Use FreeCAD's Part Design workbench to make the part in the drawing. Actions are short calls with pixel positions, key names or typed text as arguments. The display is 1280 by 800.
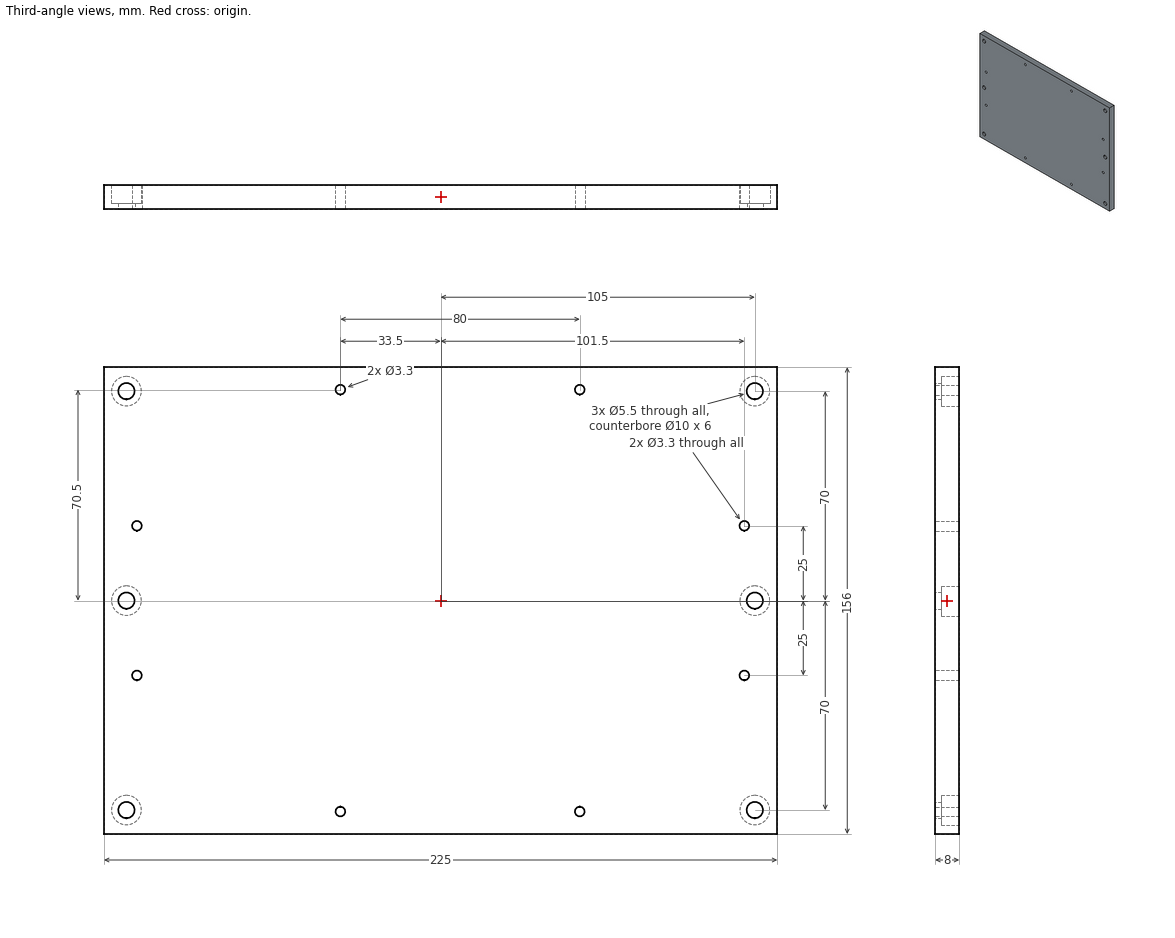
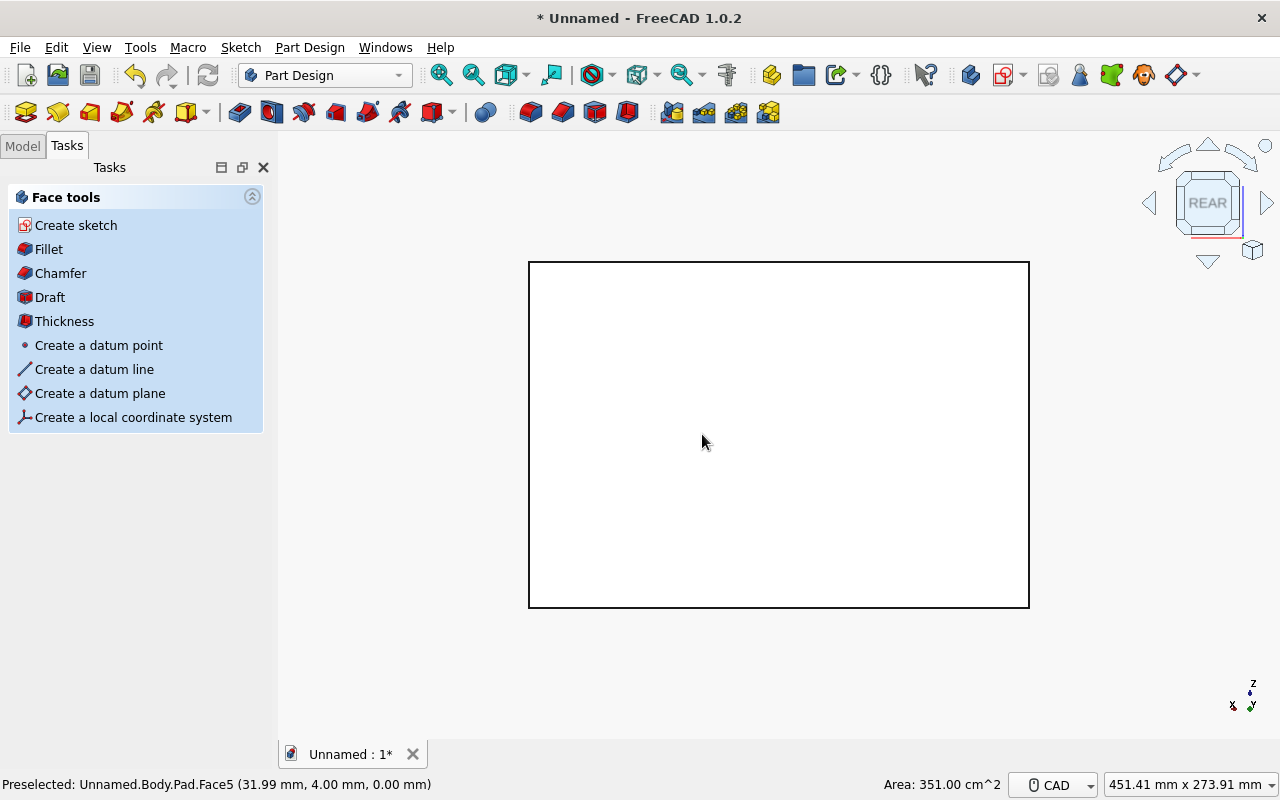
click(1004, 76)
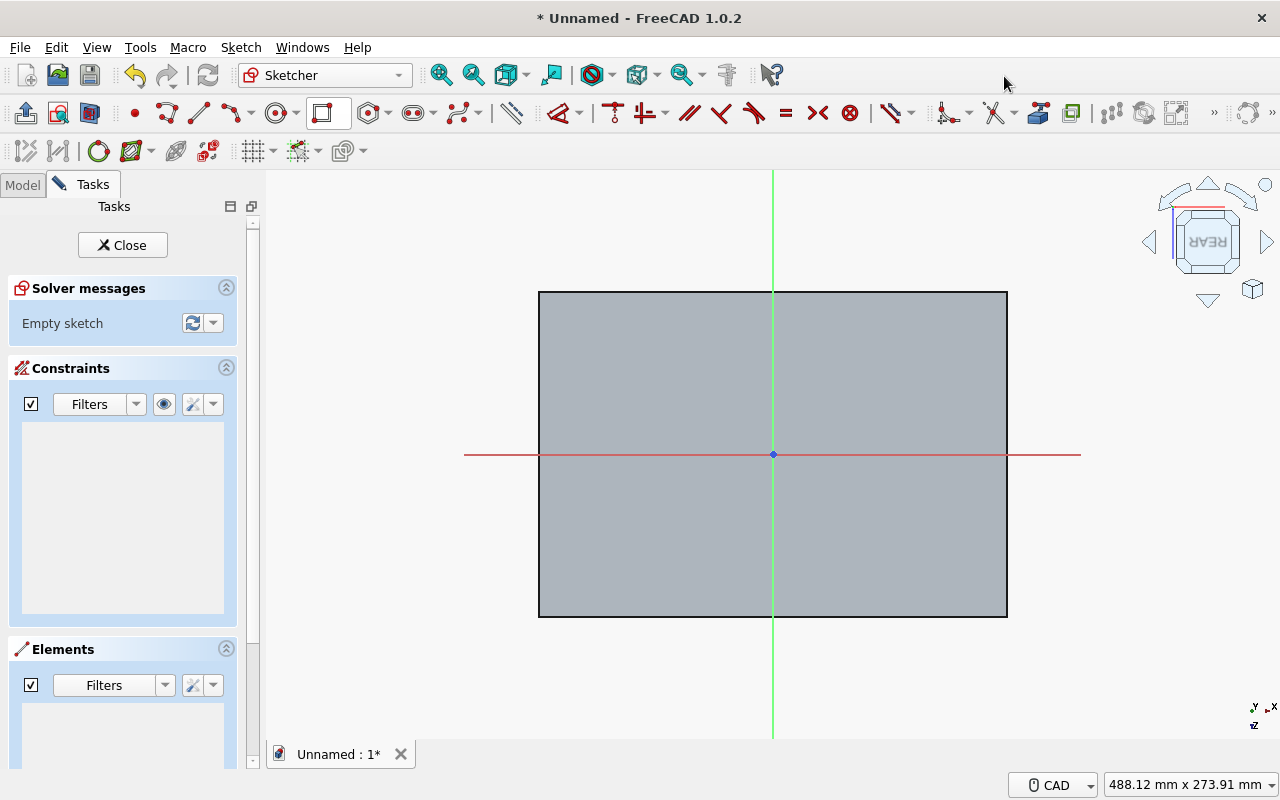
key(g)
key(c)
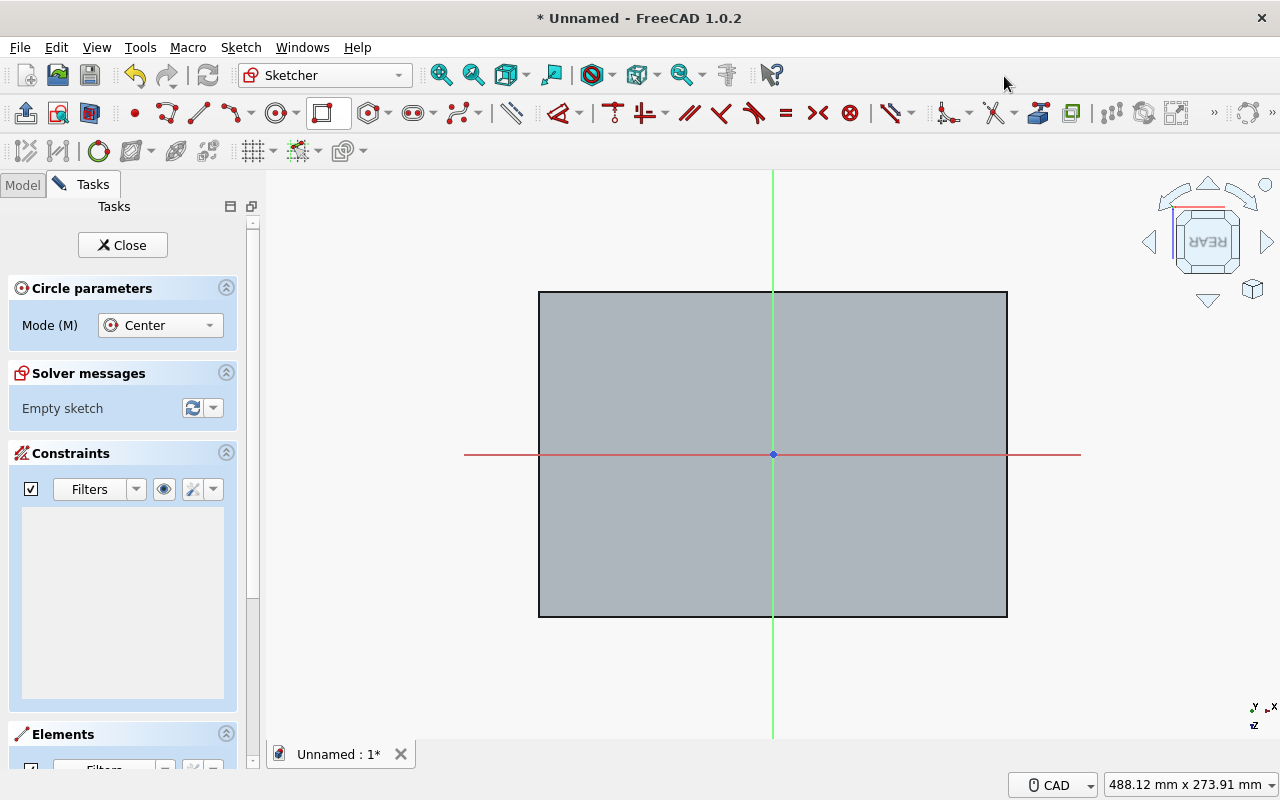
scroll(991, 600, up, 7)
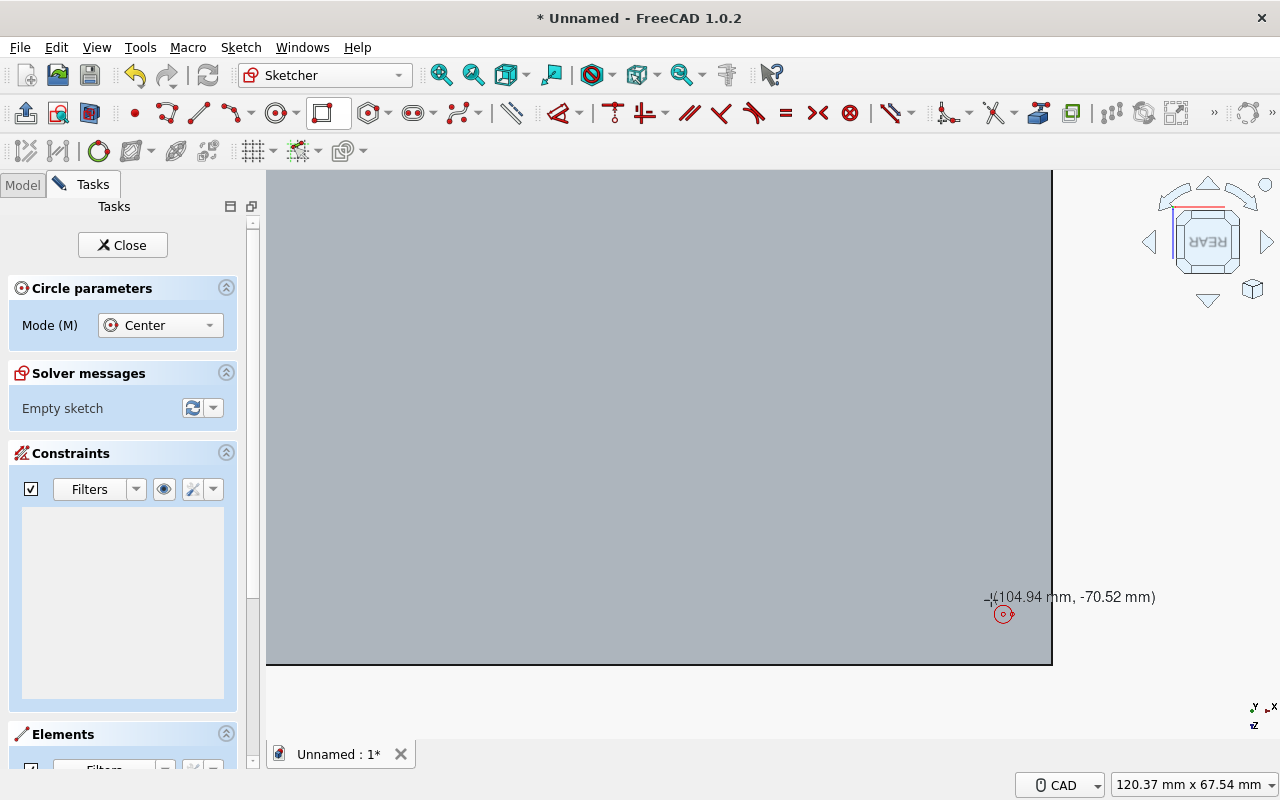
scroll(767, 647, down, 6)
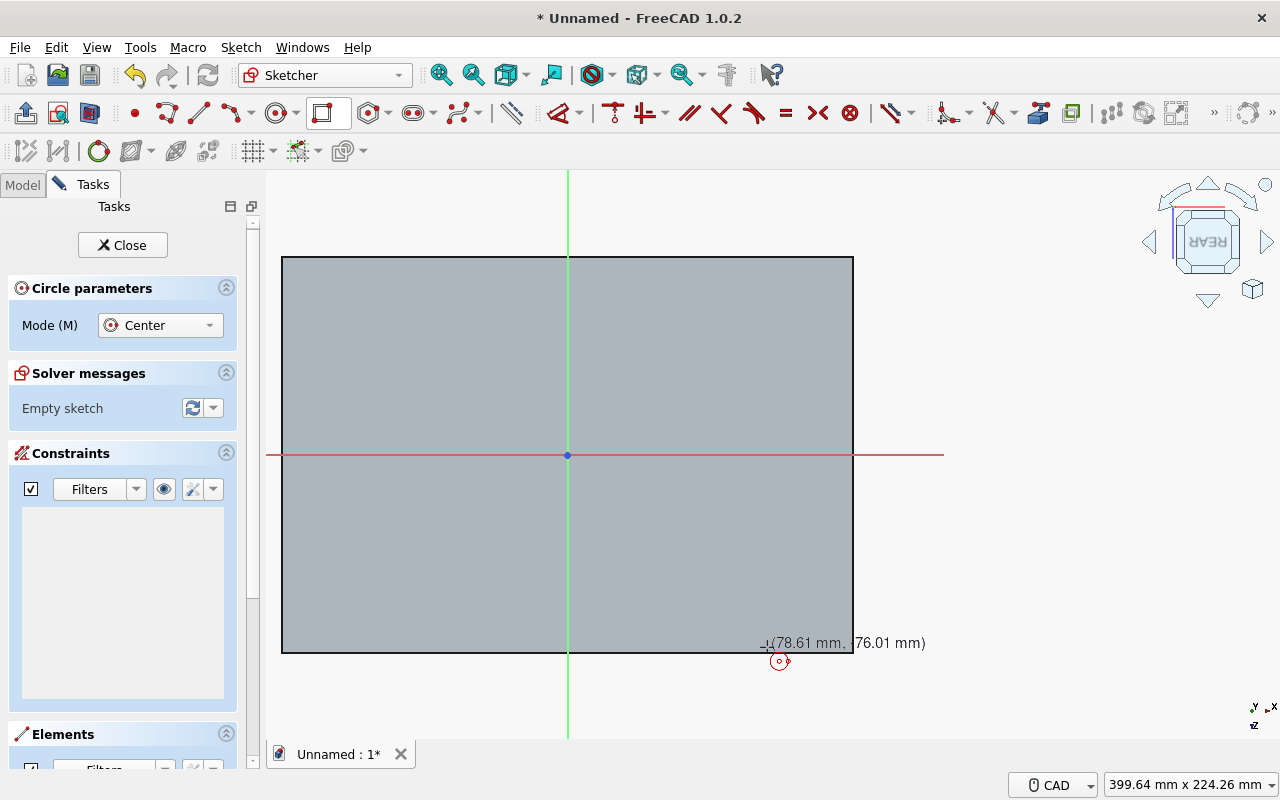
click(834, 633)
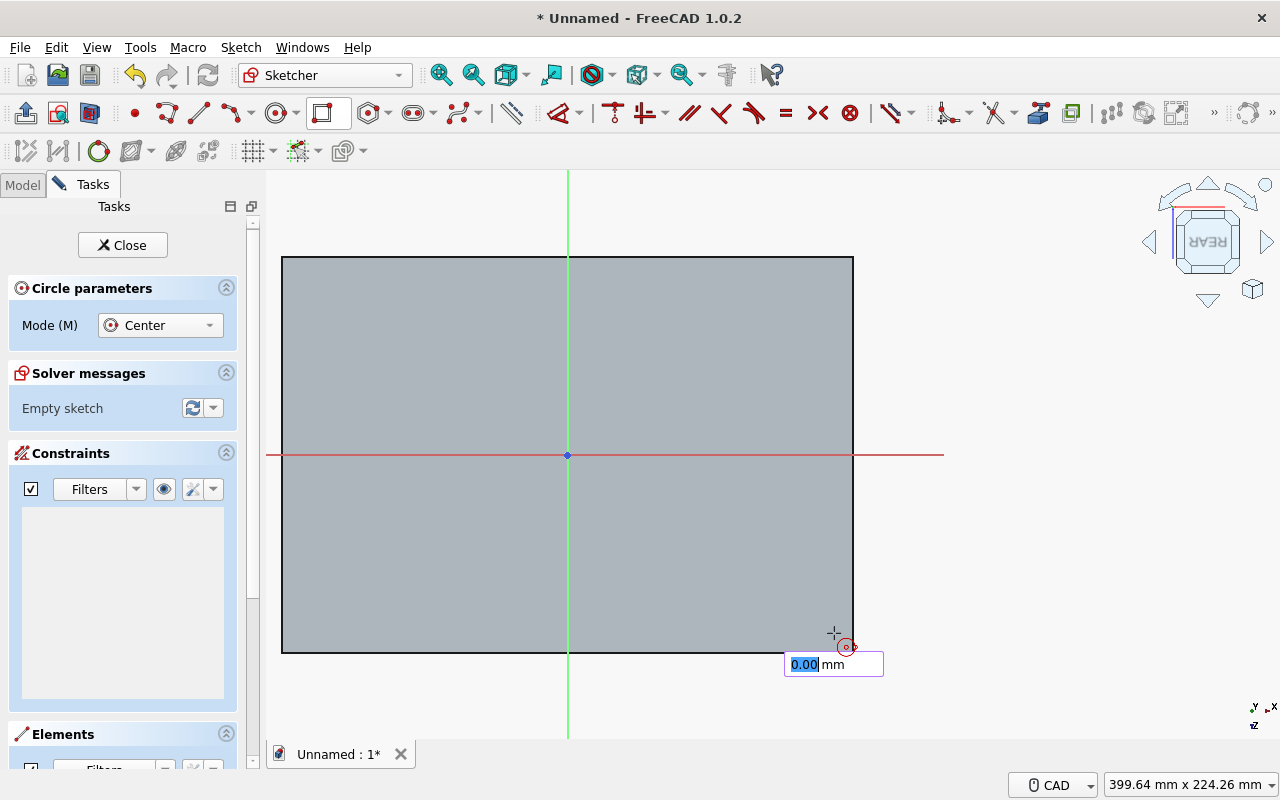
scroll(839, 628, up, 5)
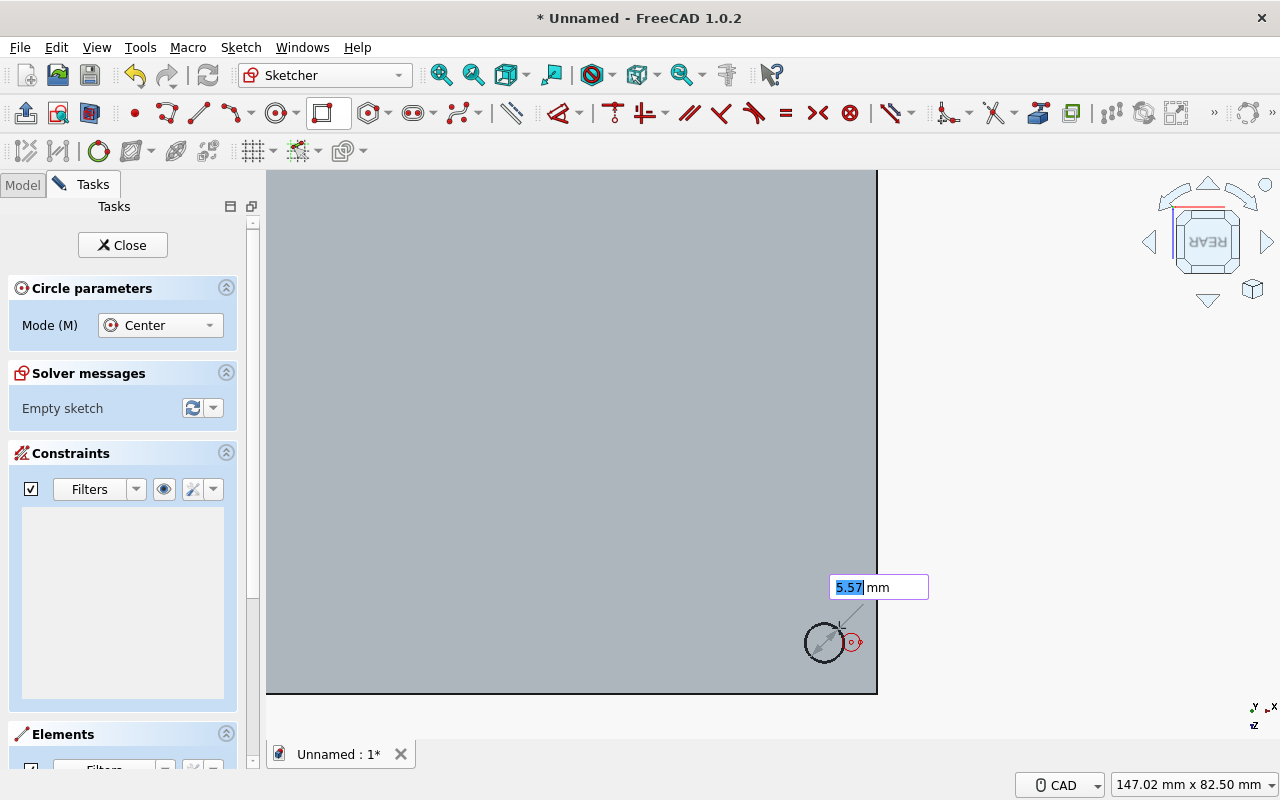
click(839, 626)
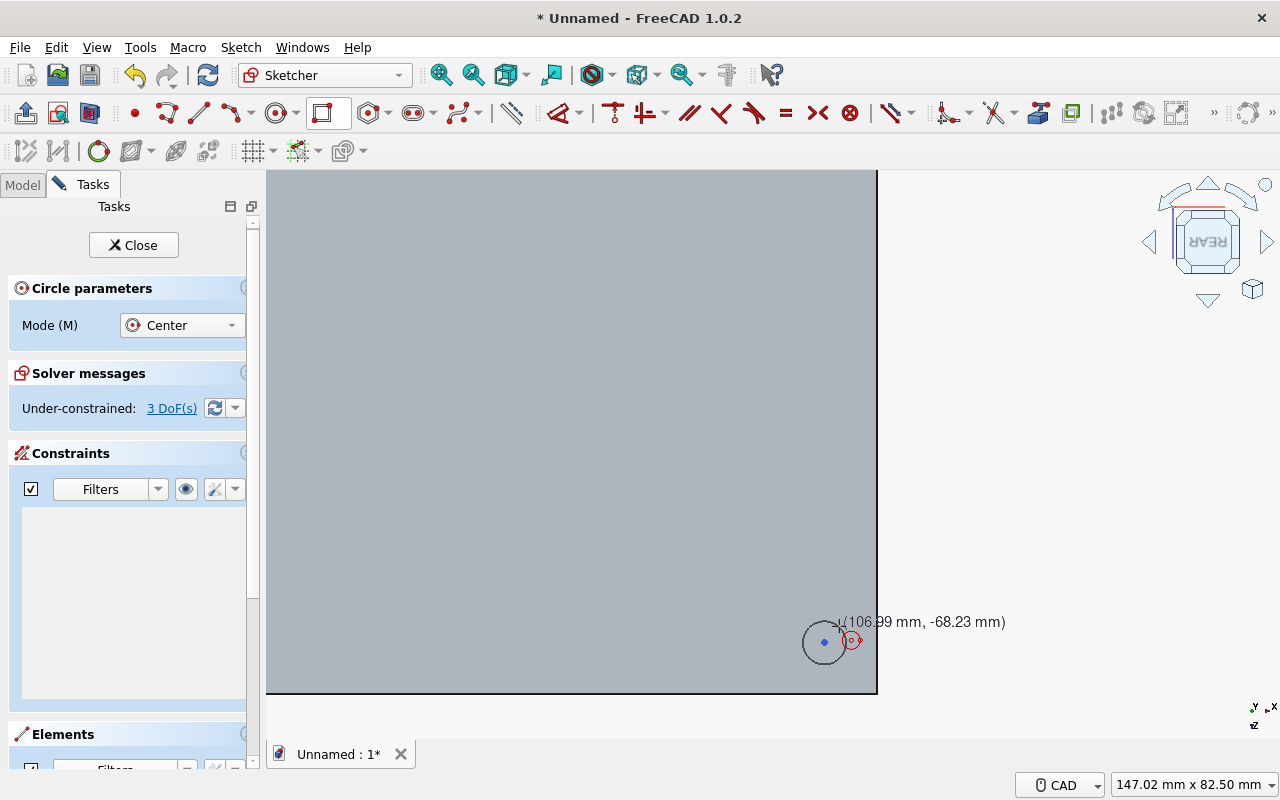
scroll(839, 628, down, 5)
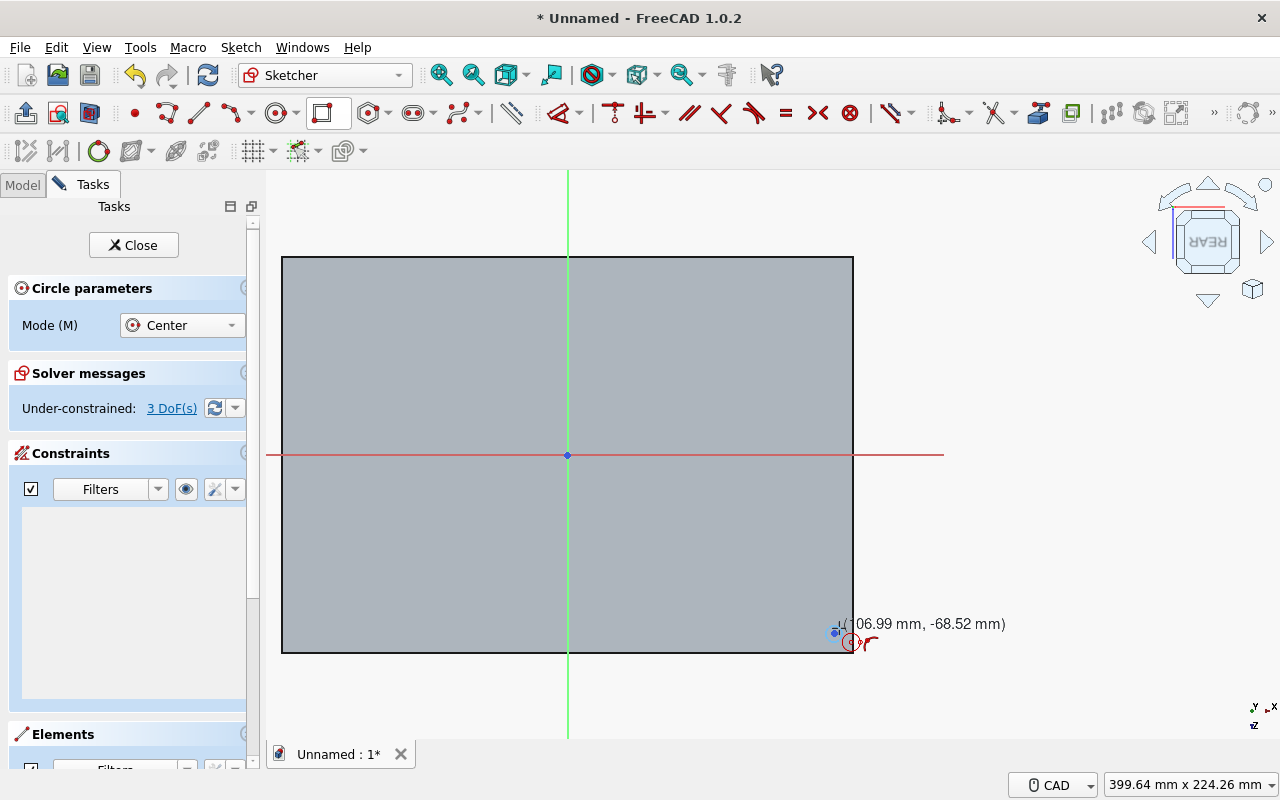
scroll(834, 455, up, 6)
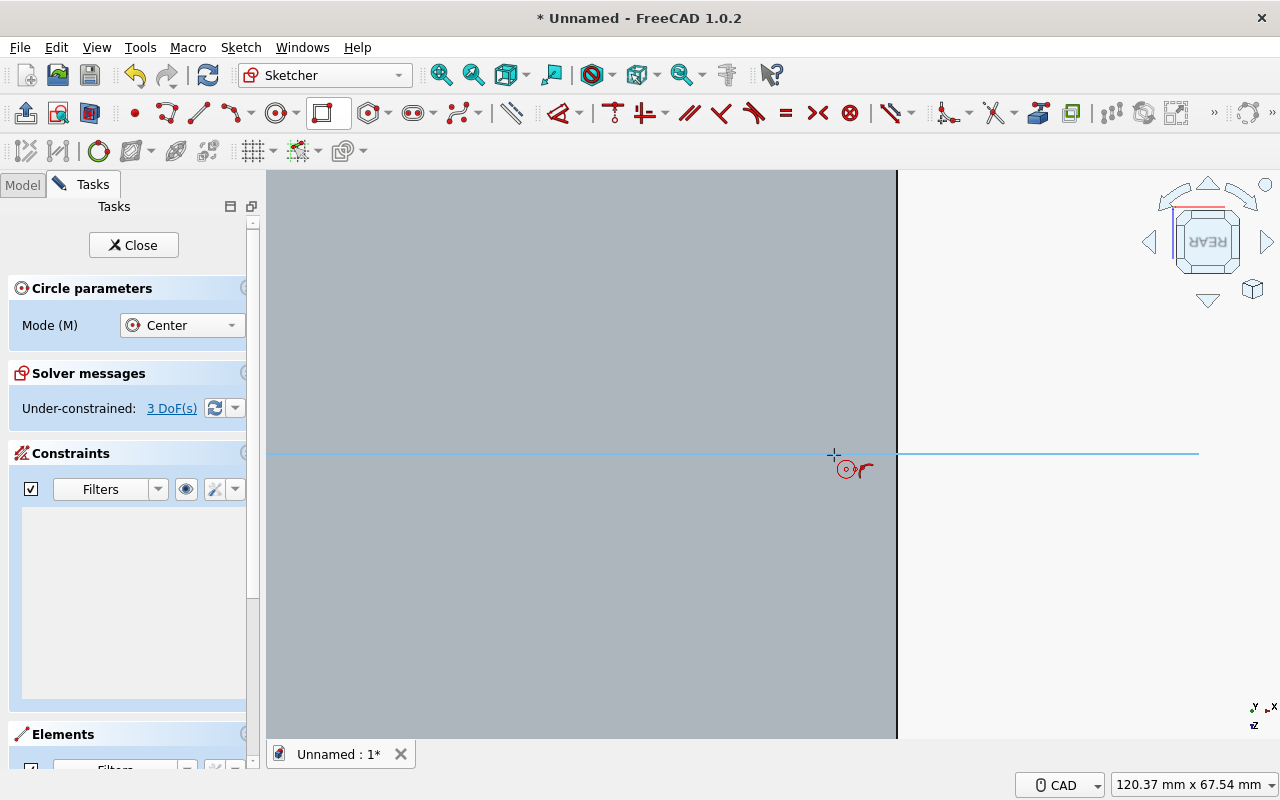
scroll(834, 455, down, 6)